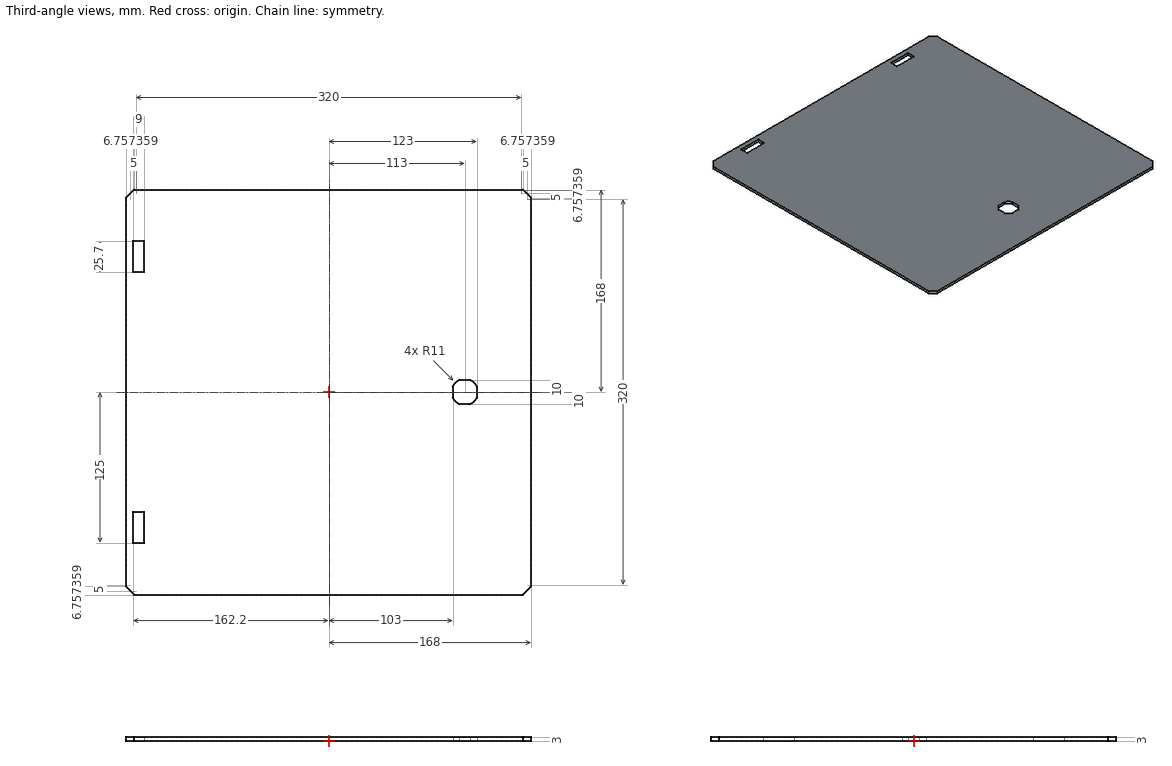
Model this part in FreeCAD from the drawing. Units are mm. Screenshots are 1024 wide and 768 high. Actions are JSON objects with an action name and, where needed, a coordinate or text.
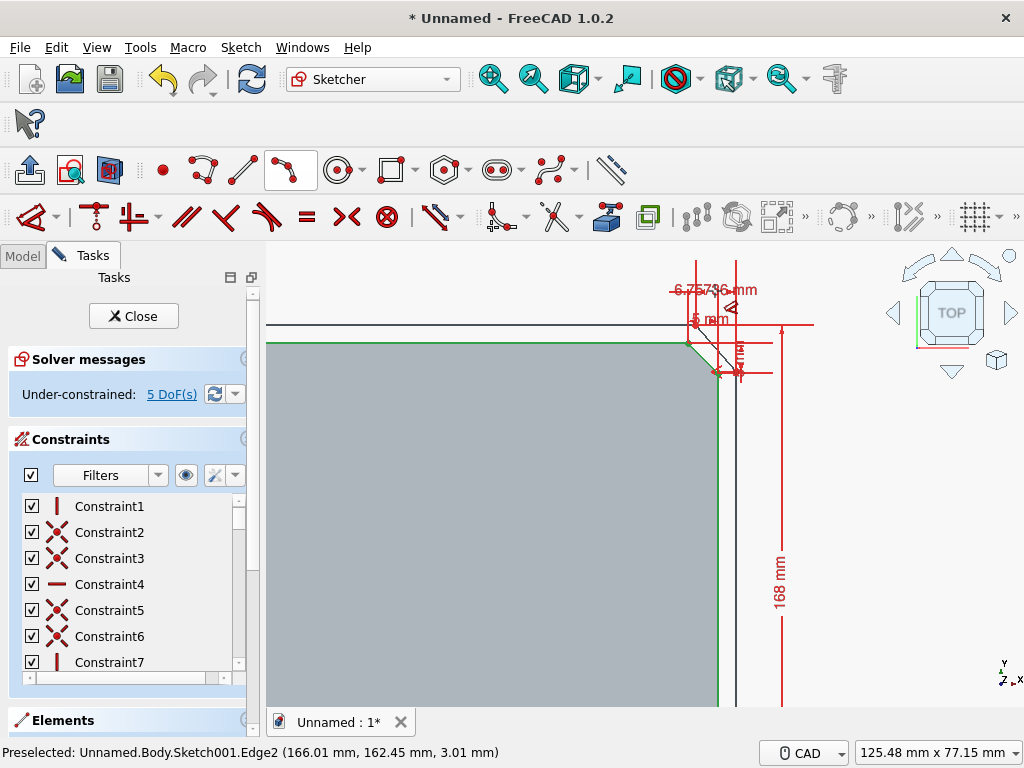
{"action": "left_click", "coordinate": [724, 358]}
{"action": "left_click", "coordinate": [662, 359]}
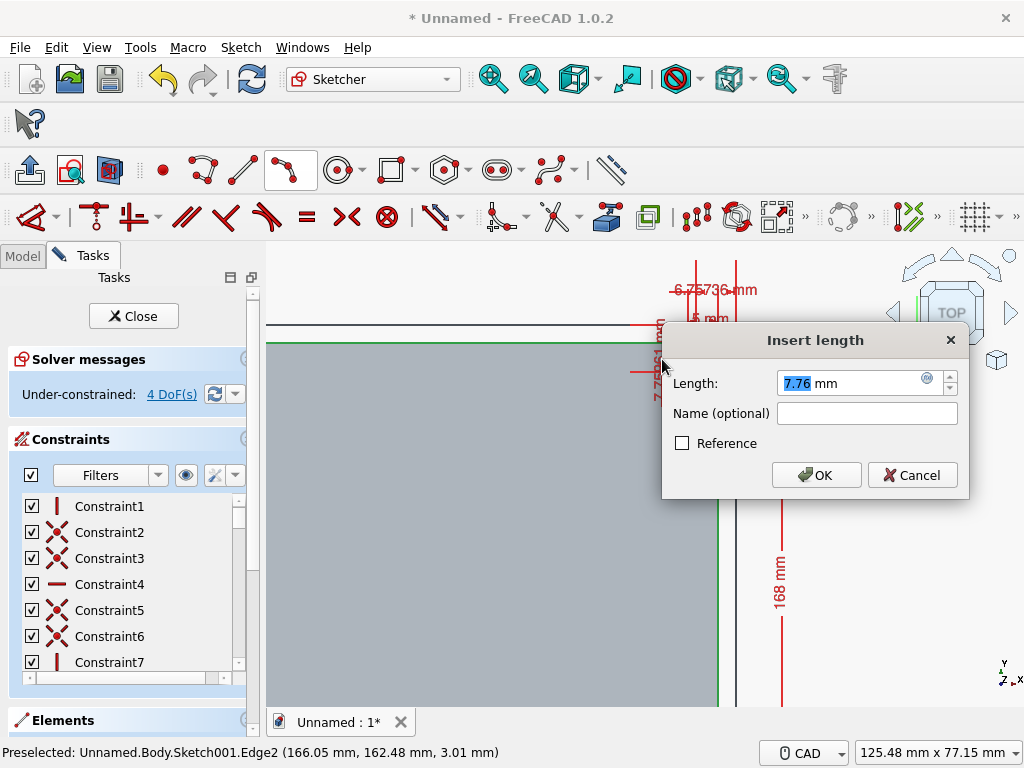
{"action": "type", "text": "6.757359"}
{"action": "key", "text": "Return"}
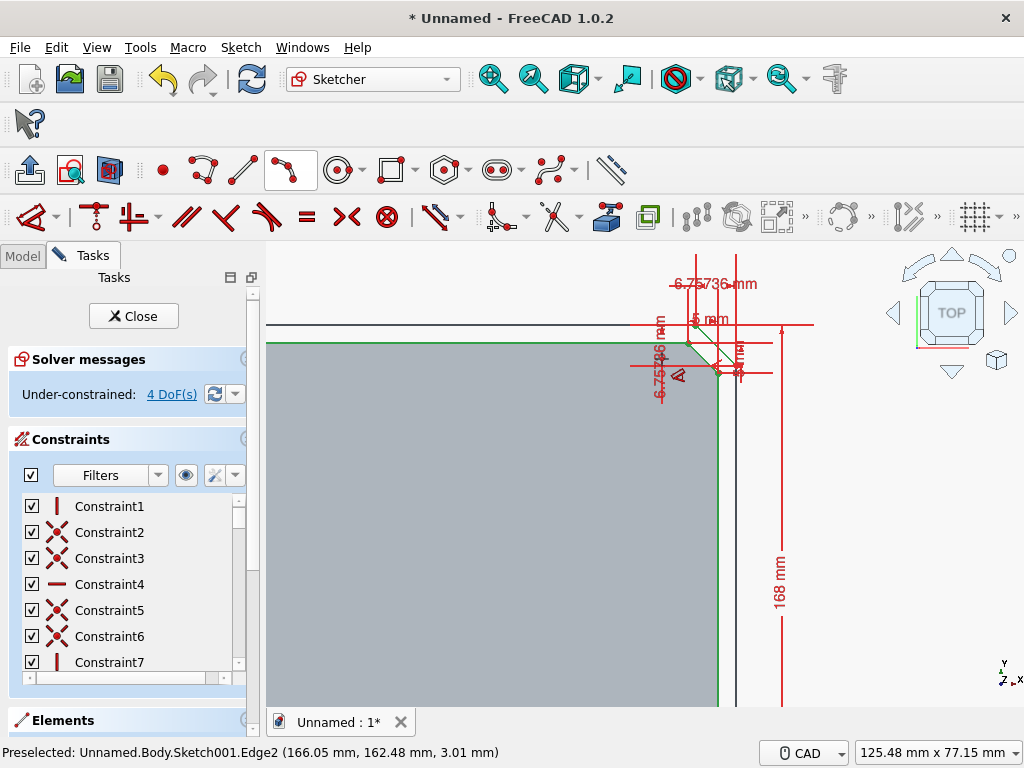
{"action": "scroll", "coordinate": [710, 338], "scroll_direction": "down", "scroll_amount": 10}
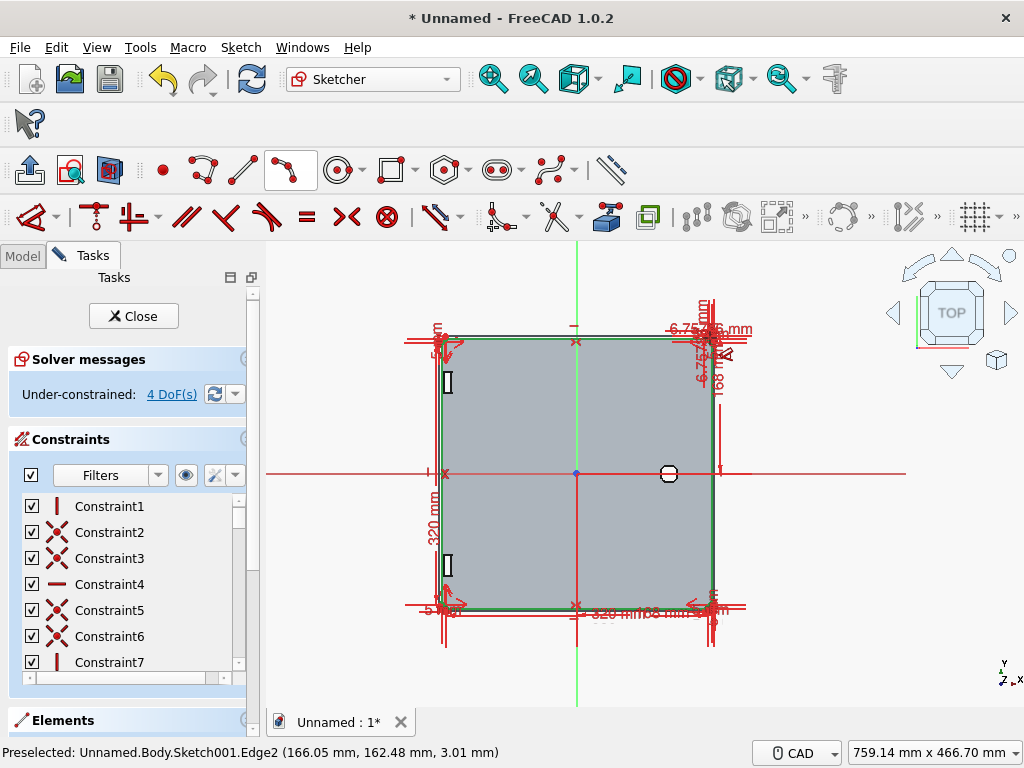
{"action": "scroll", "coordinate": [443, 338], "scroll_direction": "up", "scroll_amount": 10}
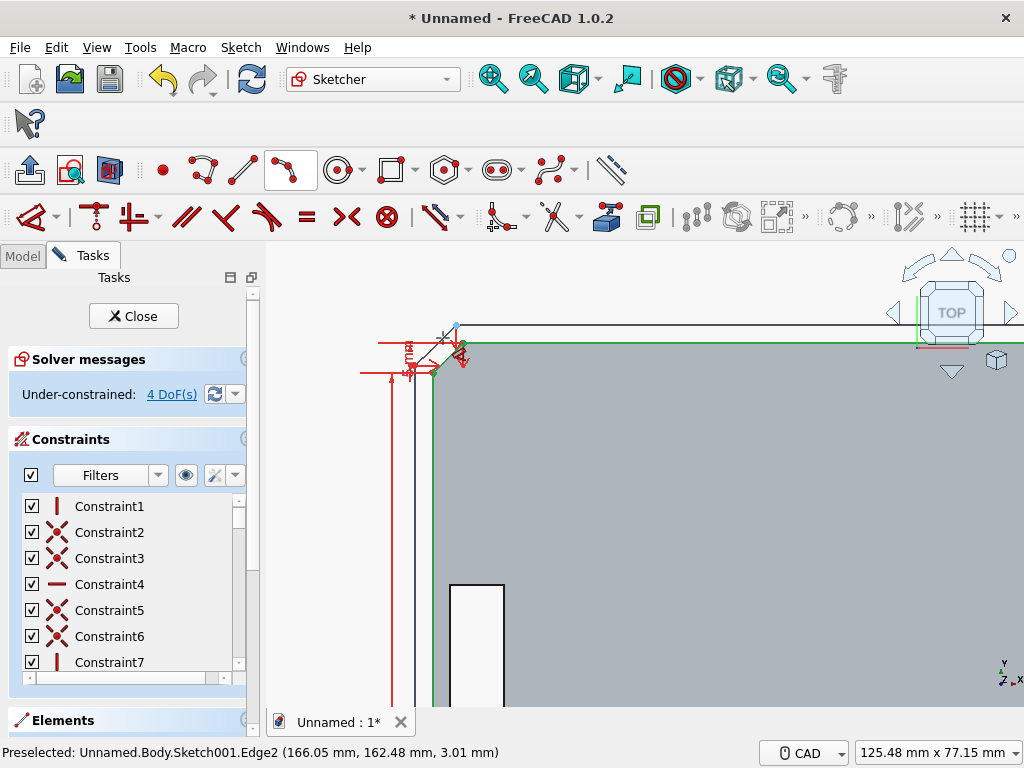
{"action": "left_click", "coordinate": [444, 337]}
{"action": "left_click", "coordinate": [436, 291]}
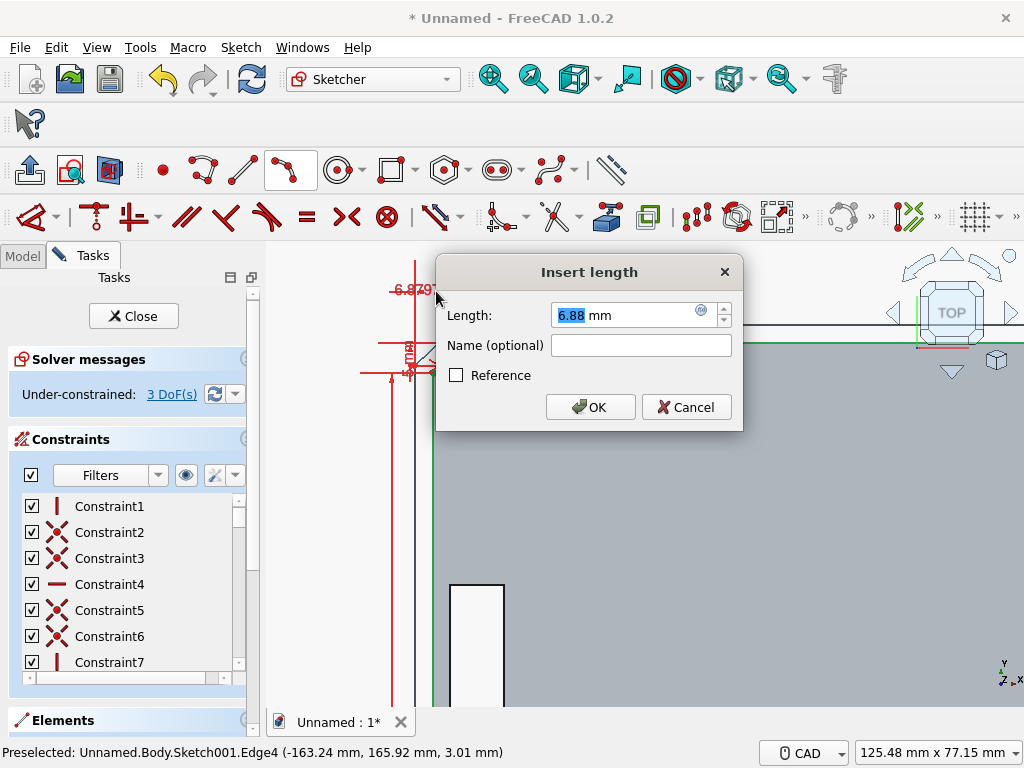
{"action": "type", "text": "6.757359"}
{"action": "key", "text": "Return"}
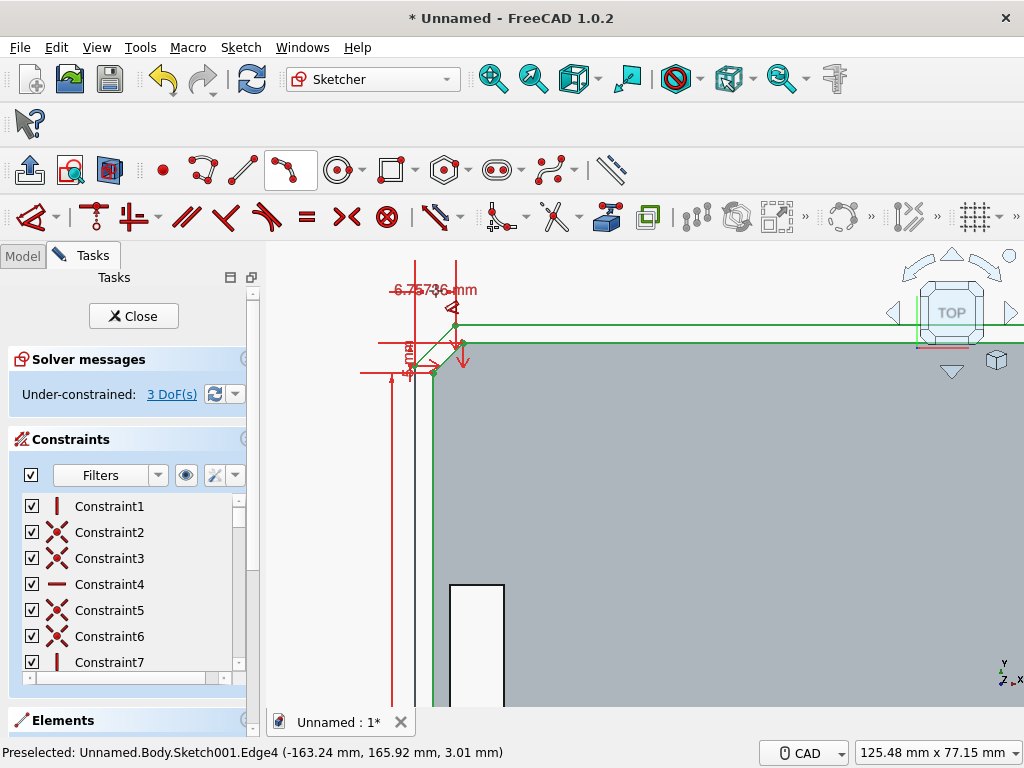
{"action": "scroll", "coordinate": [443, 338], "scroll_direction": "down", "scroll_amount": 10}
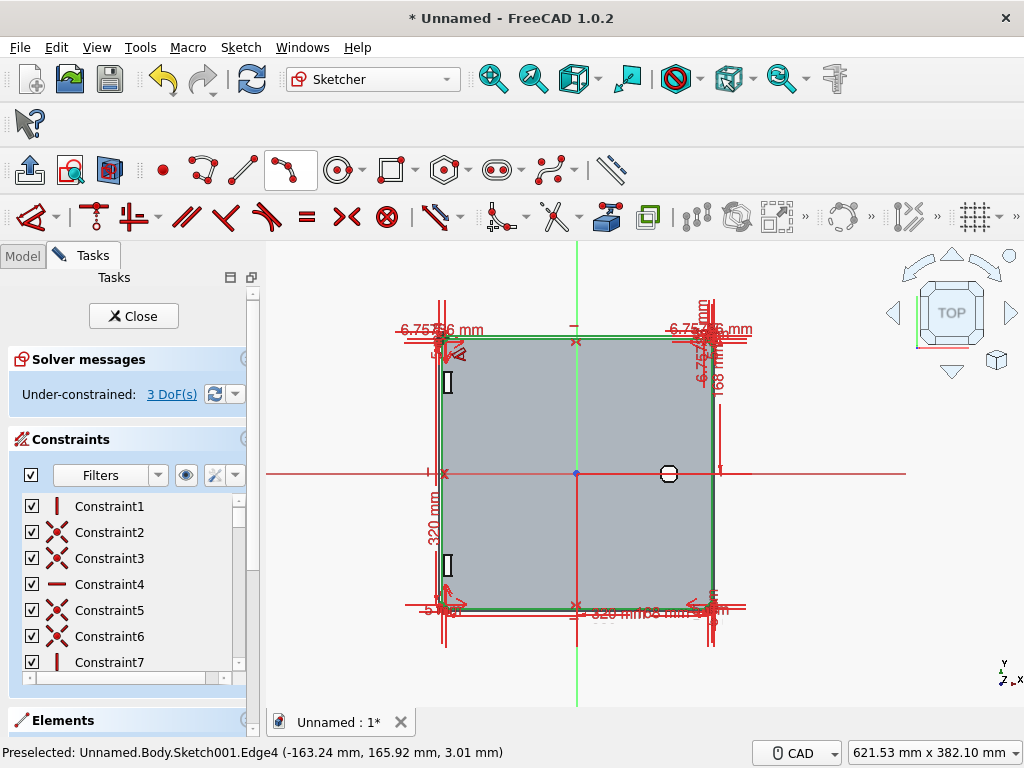
{"action": "scroll", "coordinate": [441, 608], "scroll_direction": "up", "scroll_amount": 10}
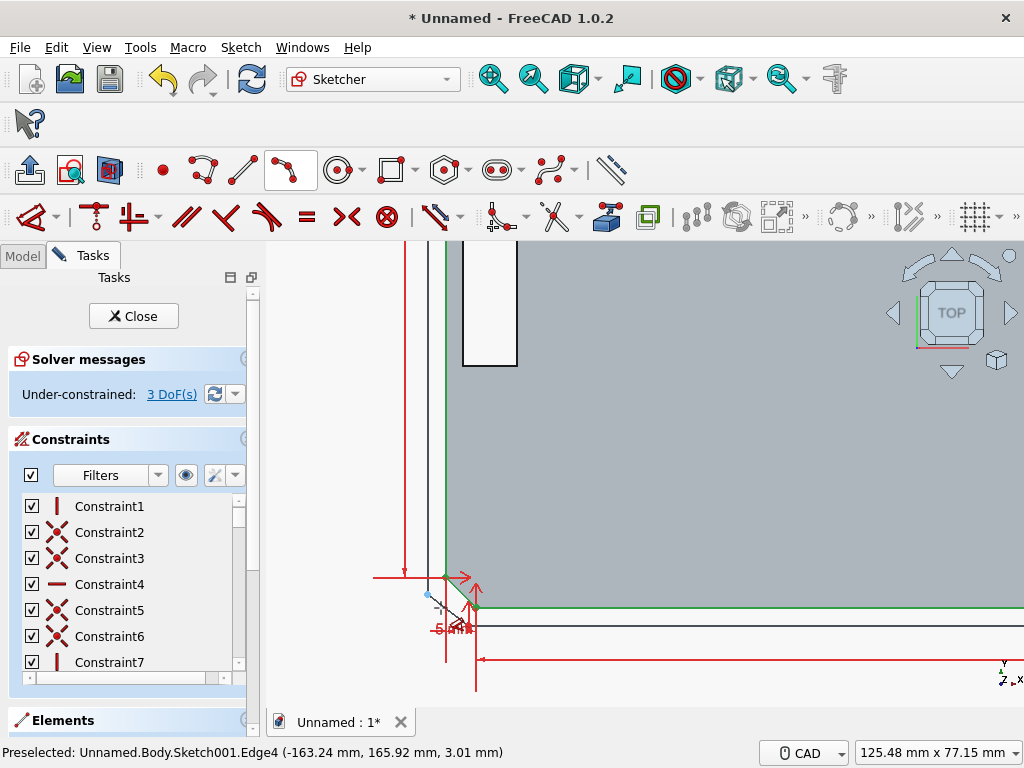
{"action": "left_click", "coordinate": [440, 604]}
{"action": "left_click", "coordinate": [394, 603]}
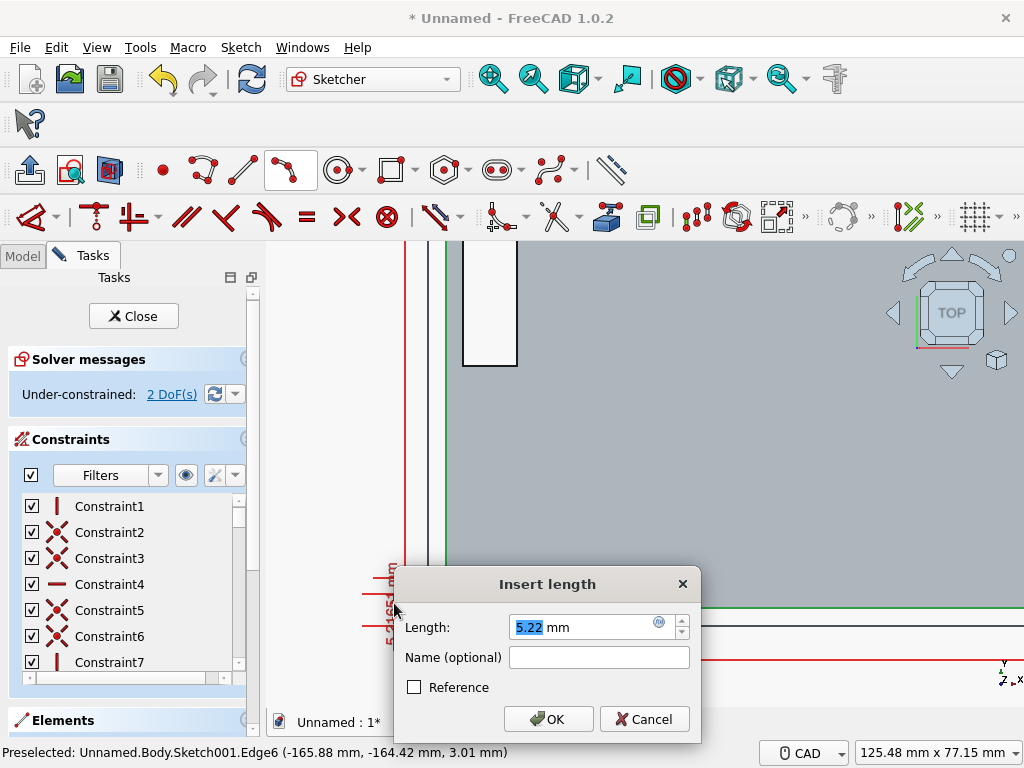
{"action": "type", "text": "6.757359"}
{"action": "key", "text": "Return"}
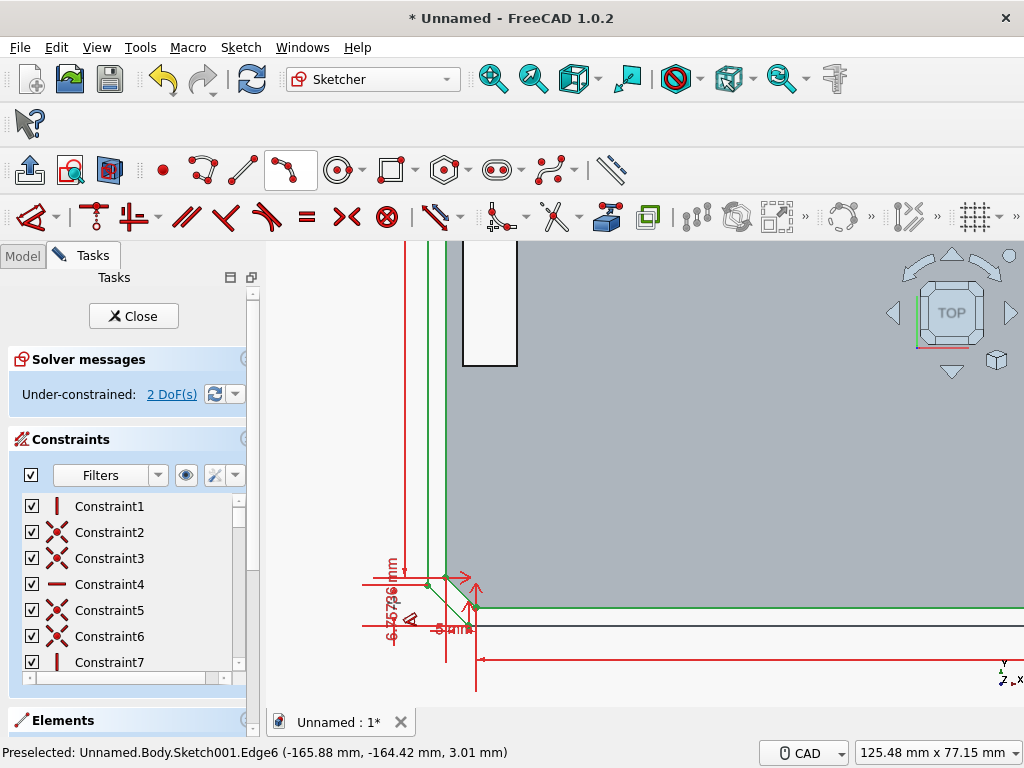
{"action": "scroll", "coordinate": [441, 609], "scroll_direction": "down", "scroll_amount": 10}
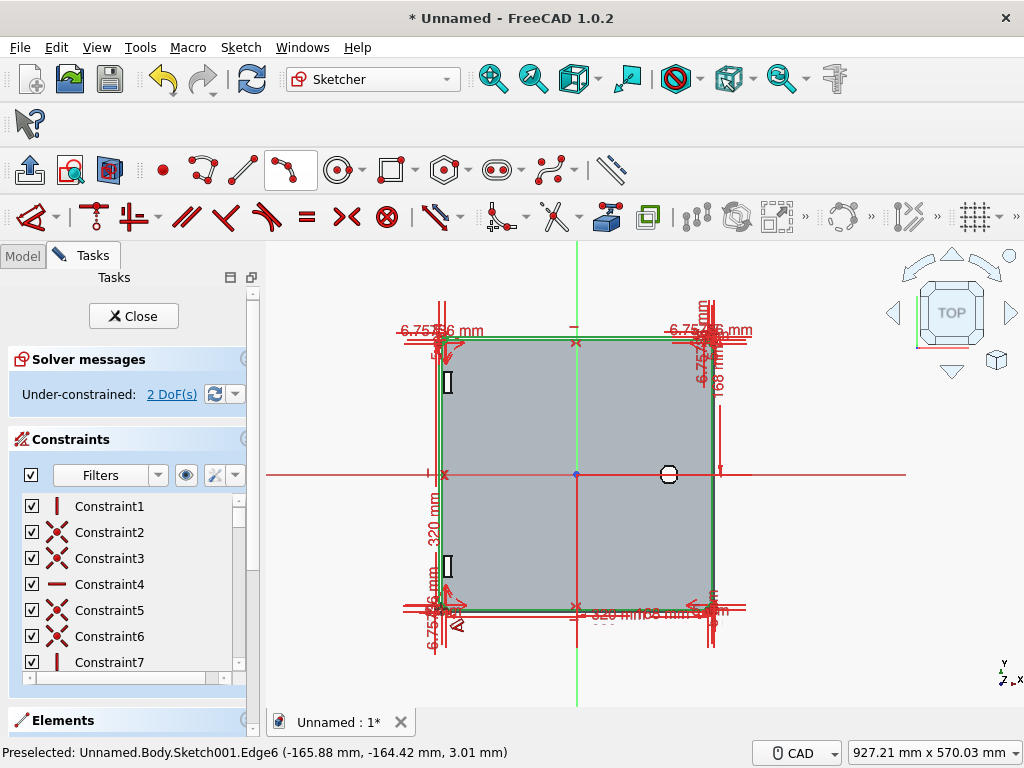
{"action": "scroll", "coordinate": [710, 611], "scroll_direction": "up", "scroll_amount": 10}